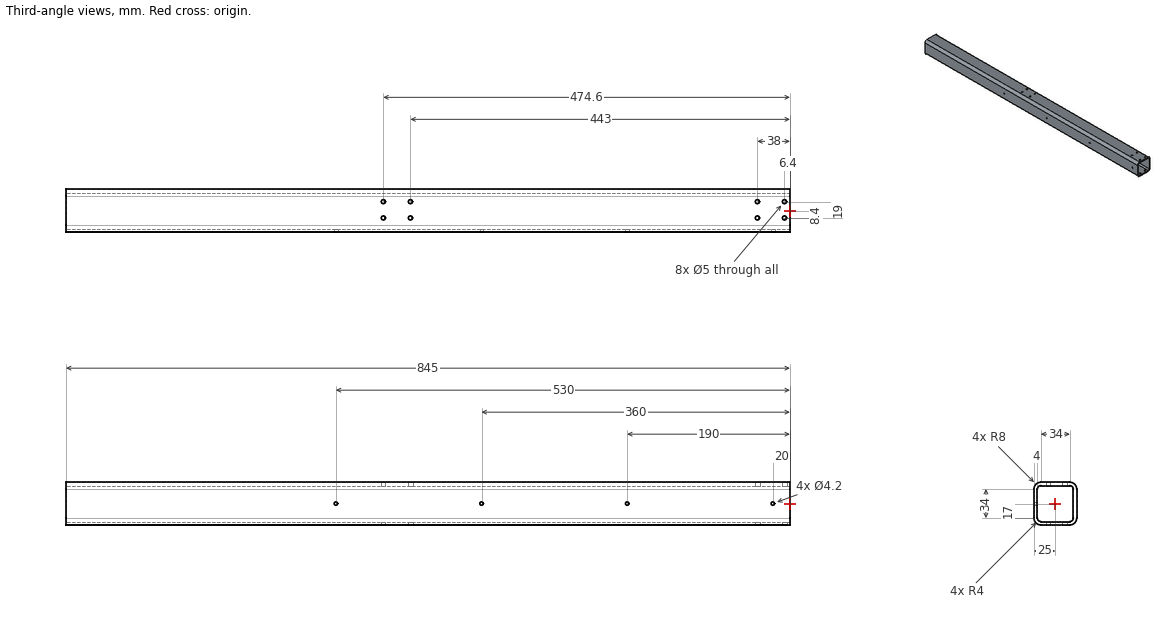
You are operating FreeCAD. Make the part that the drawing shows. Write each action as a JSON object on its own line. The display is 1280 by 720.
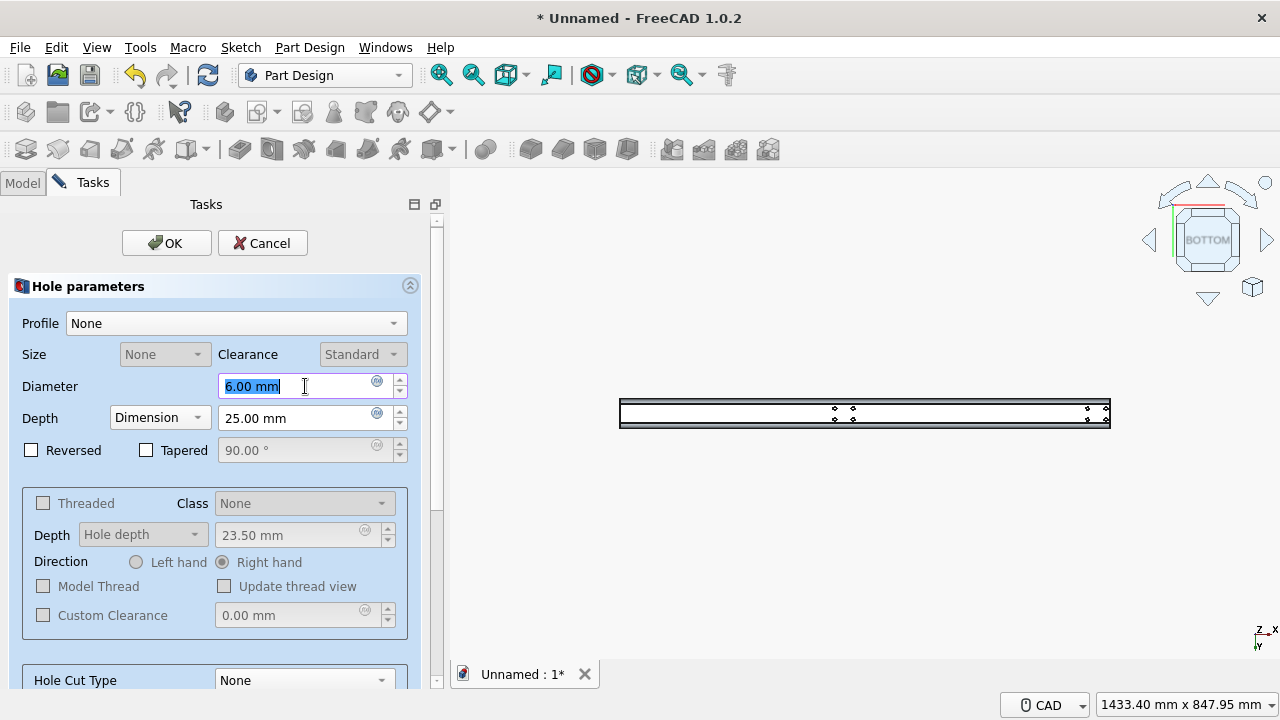
{"action": "type", "text": "5"}
{"action": "key", "text": "Tab"}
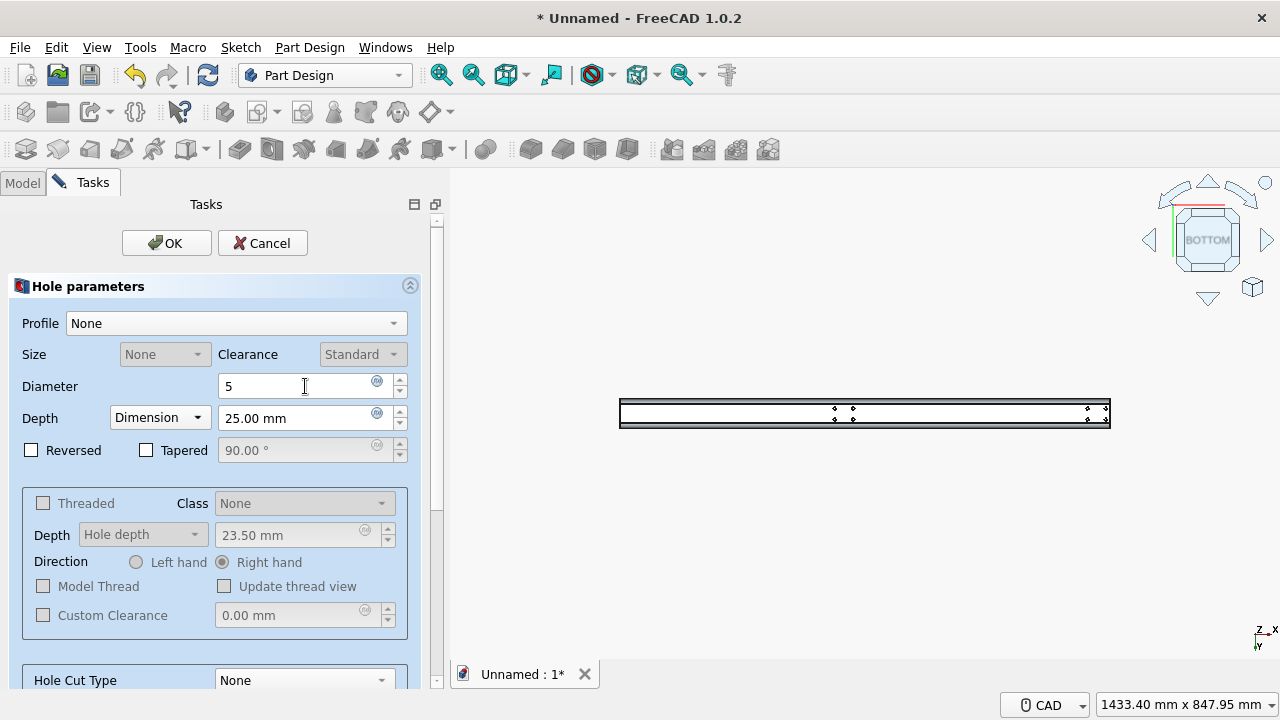
{"action": "left_click", "coordinate": [161, 418]}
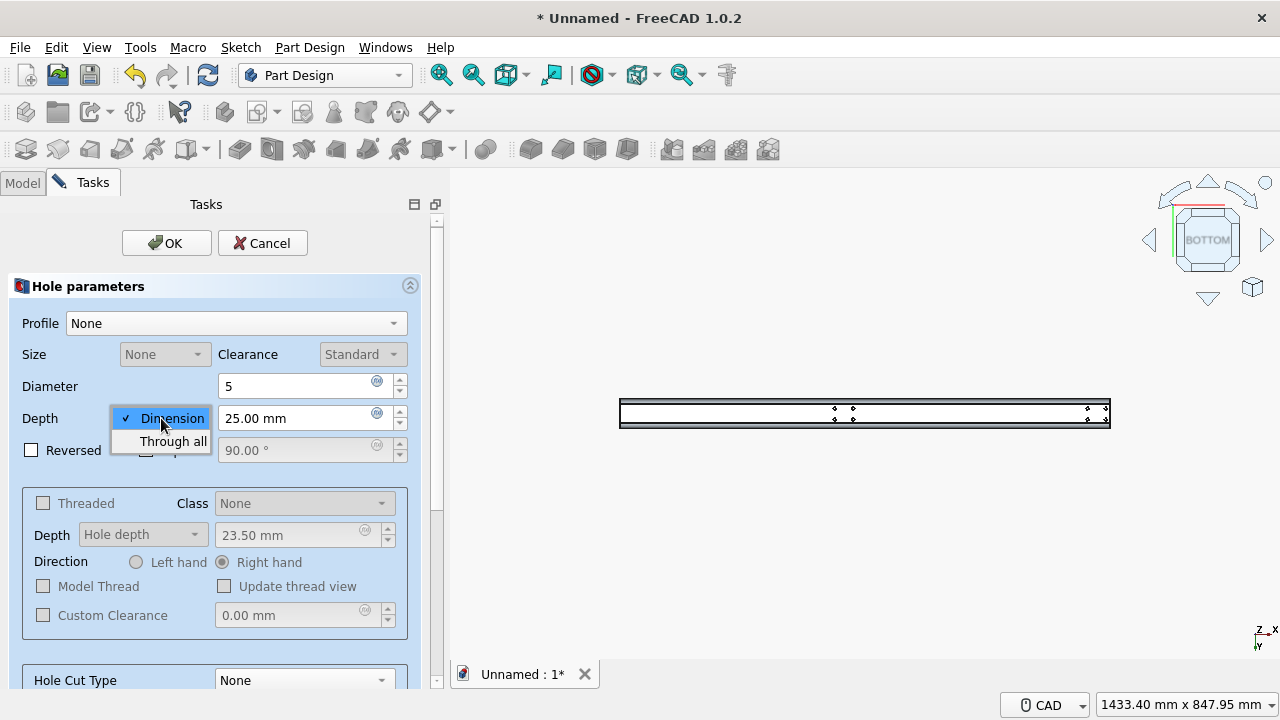
{"action": "left_click", "coordinate": [160, 442]}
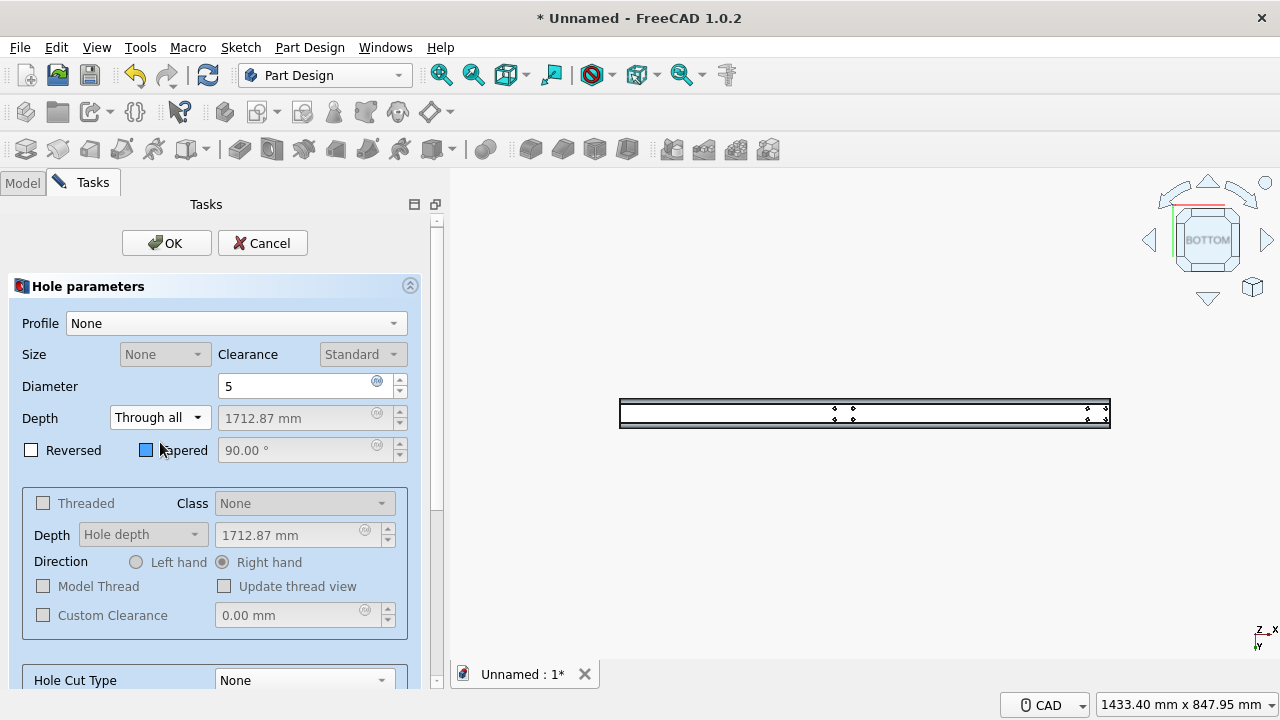
{"action": "left_click", "coordinate": [167, 243]}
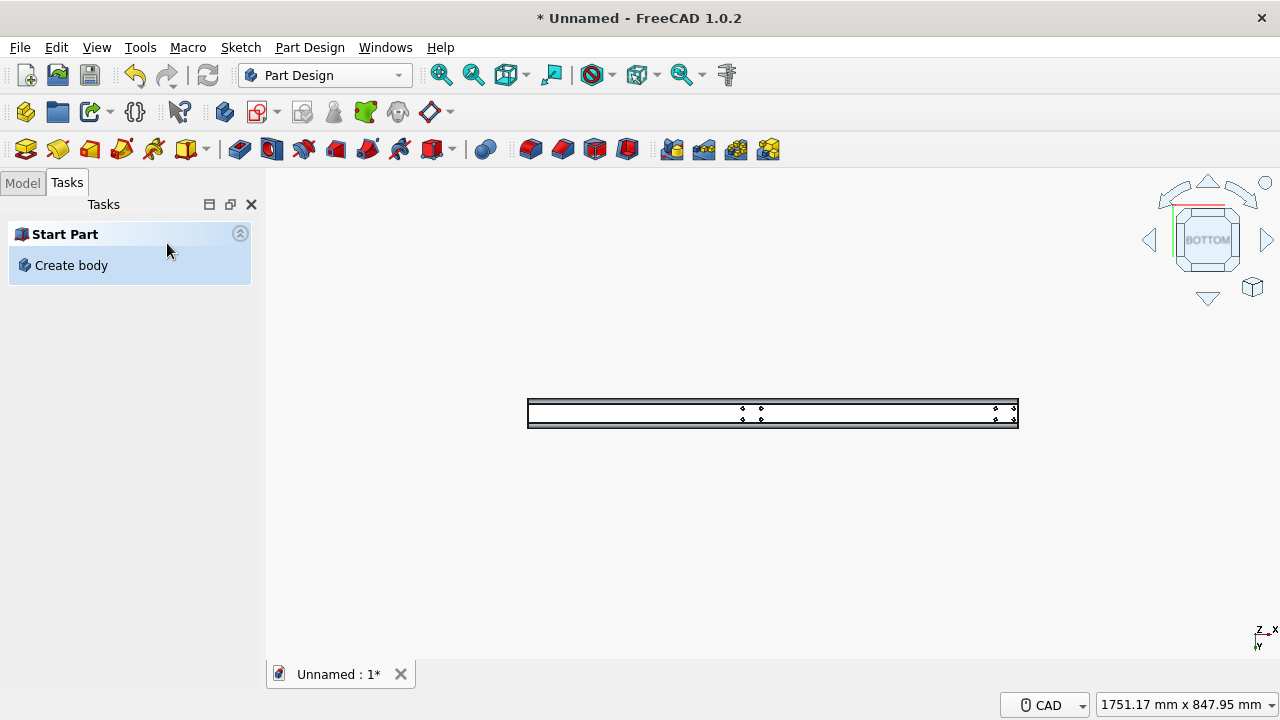
{"action": "key", "text": "0"}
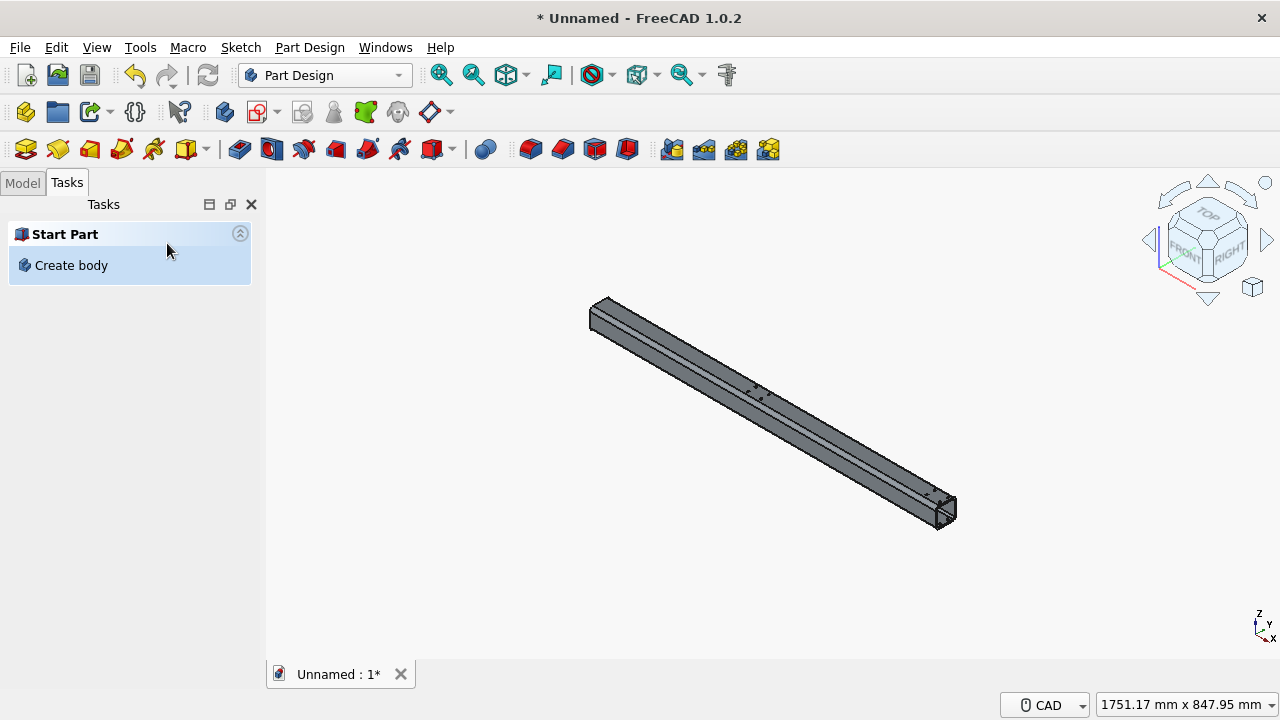
{"action": "key", "text": "1"}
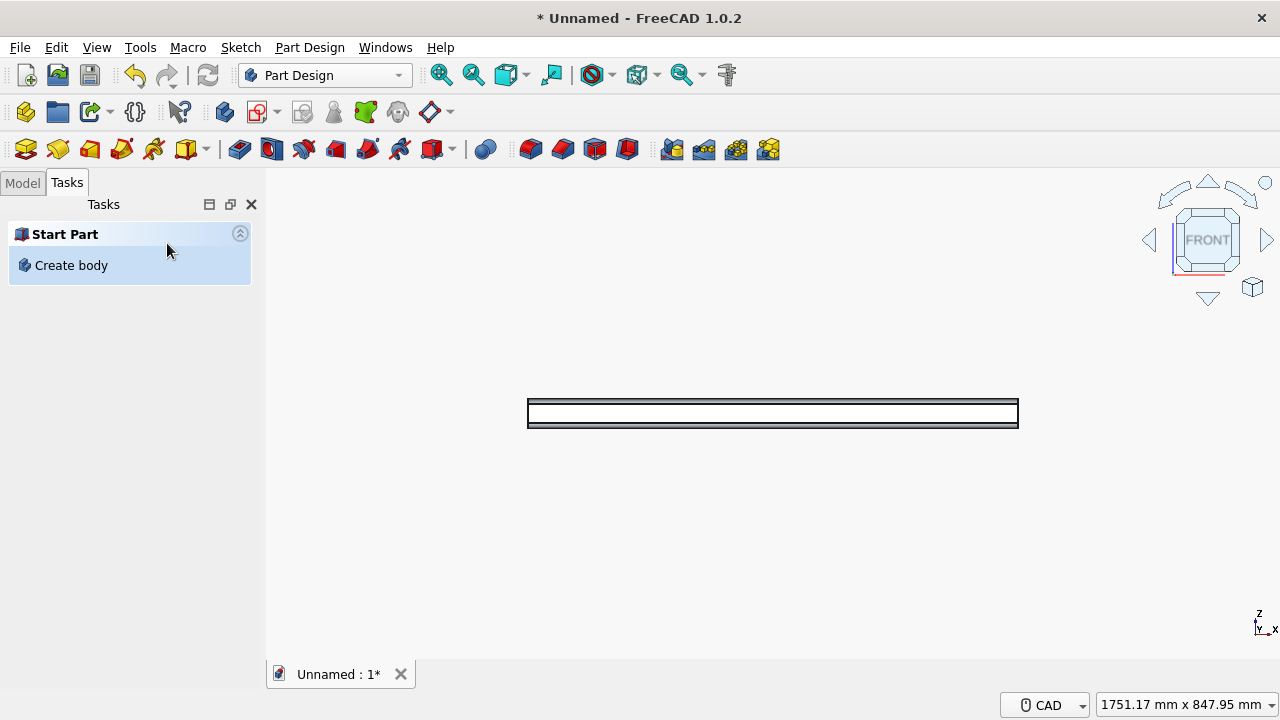
{"action": "left_click", "coordinate": [773, 412]}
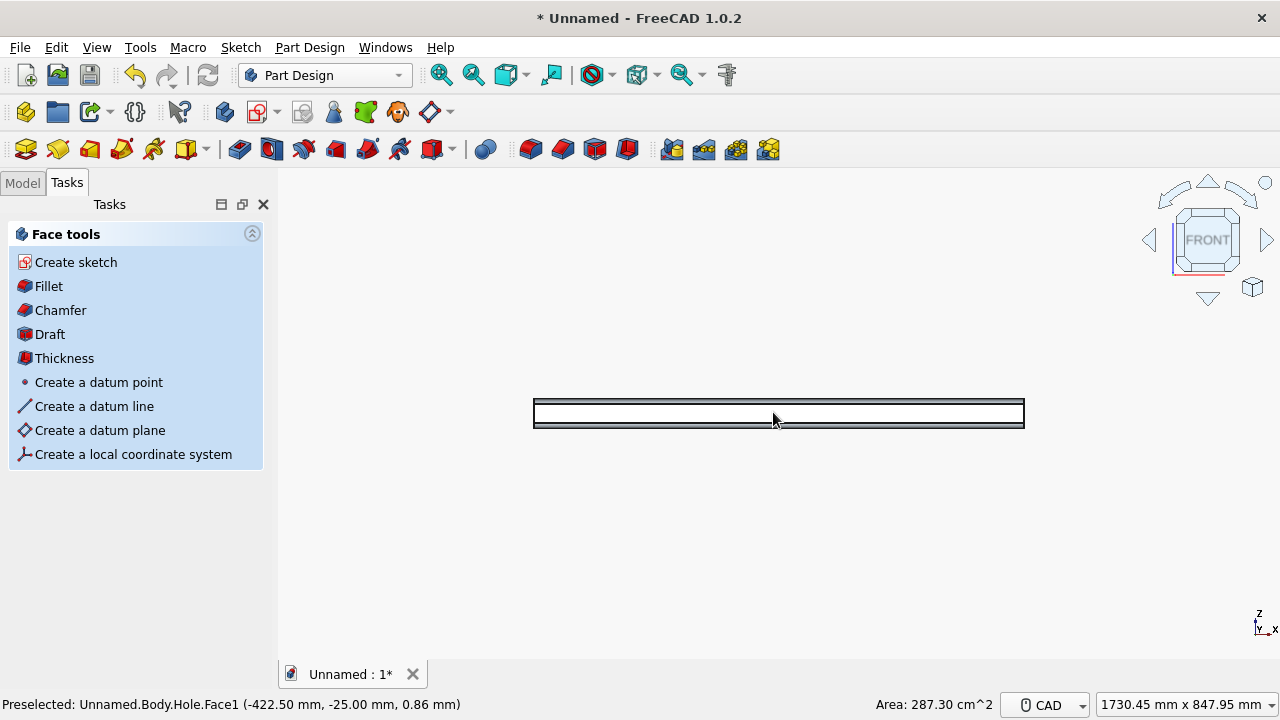
{"action": "left_click", "coordinate": [258, 112]}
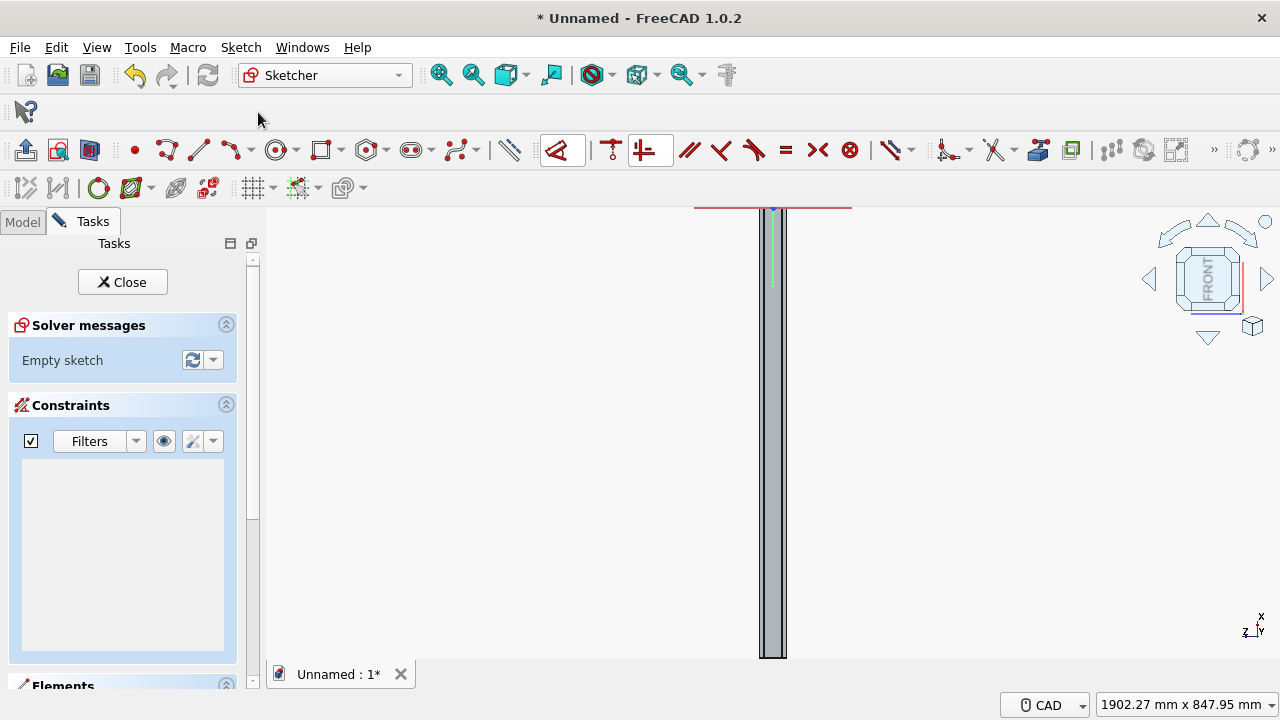
{"action": "scroll", "coordinate": [395, 631], "scroll_direction": "down", "scroll_amount": 1}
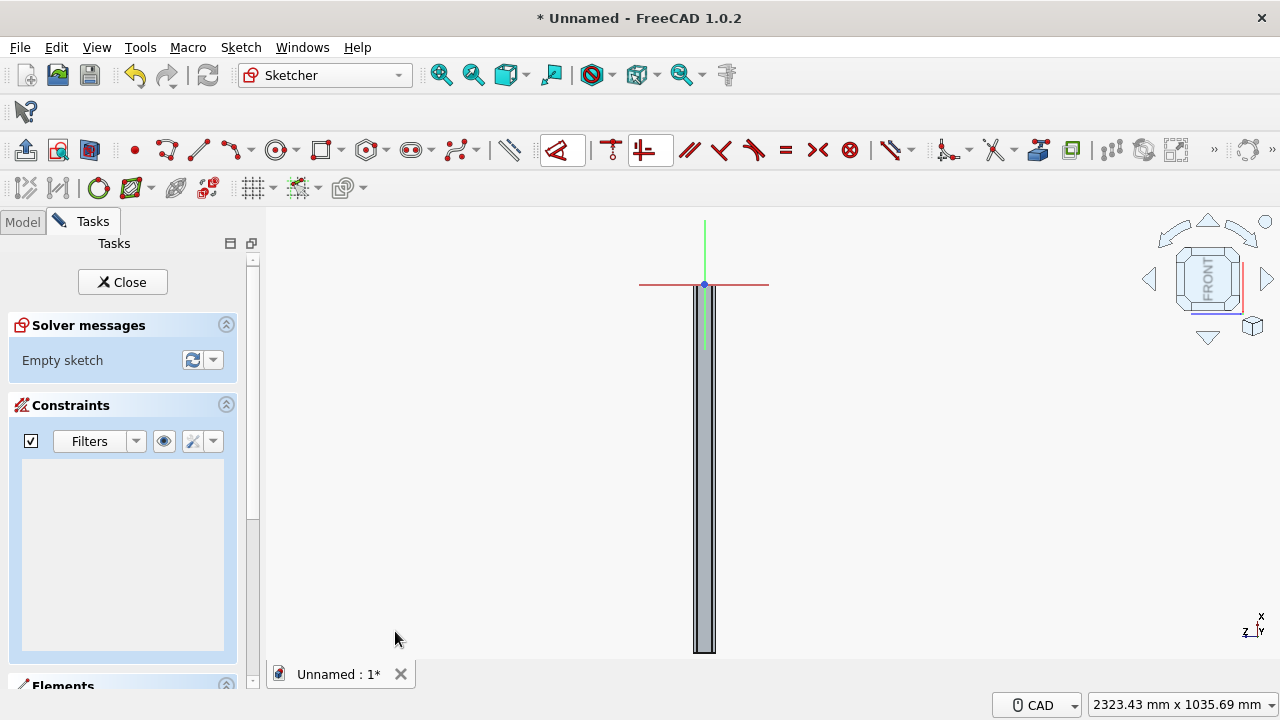
{"action": "left_click", "coordinate": [276, 150]}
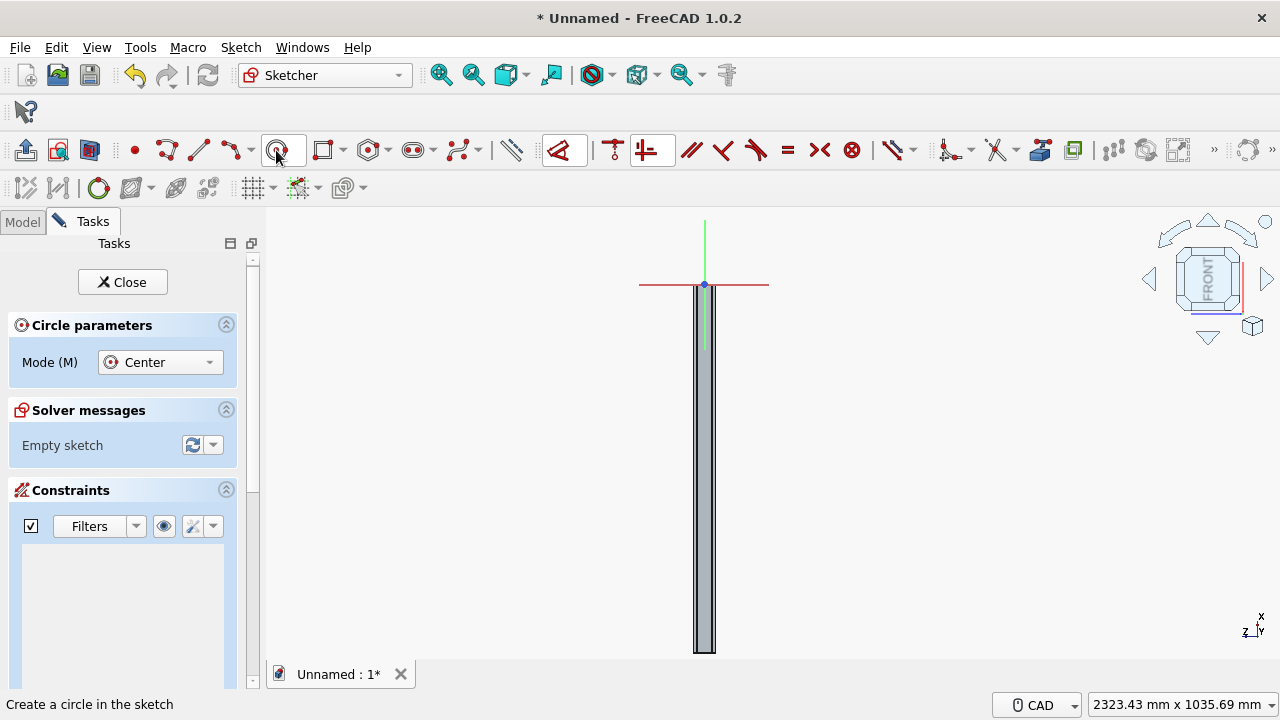
{"action": "scroll", "coordinate": [705, 293], "scroll_direction": "up", "scroll_amount": 17}